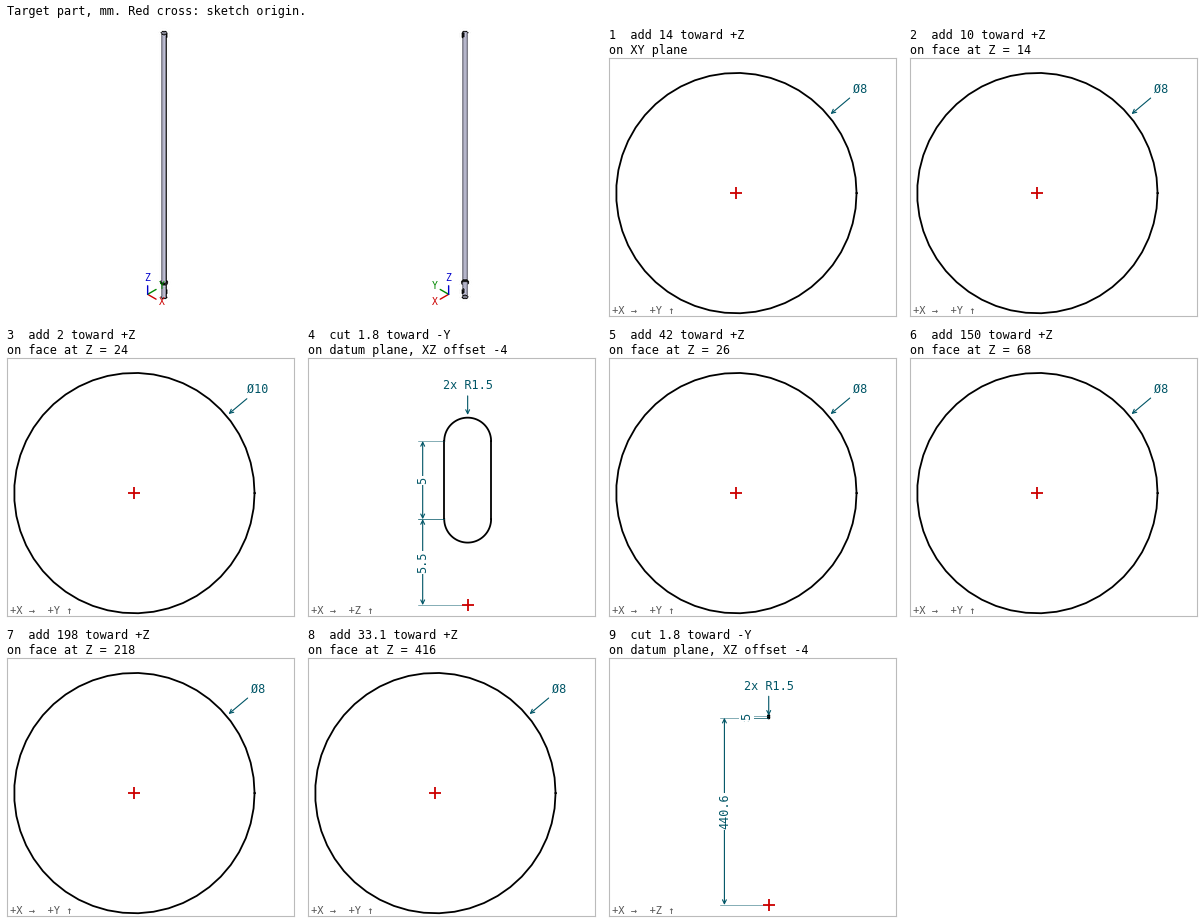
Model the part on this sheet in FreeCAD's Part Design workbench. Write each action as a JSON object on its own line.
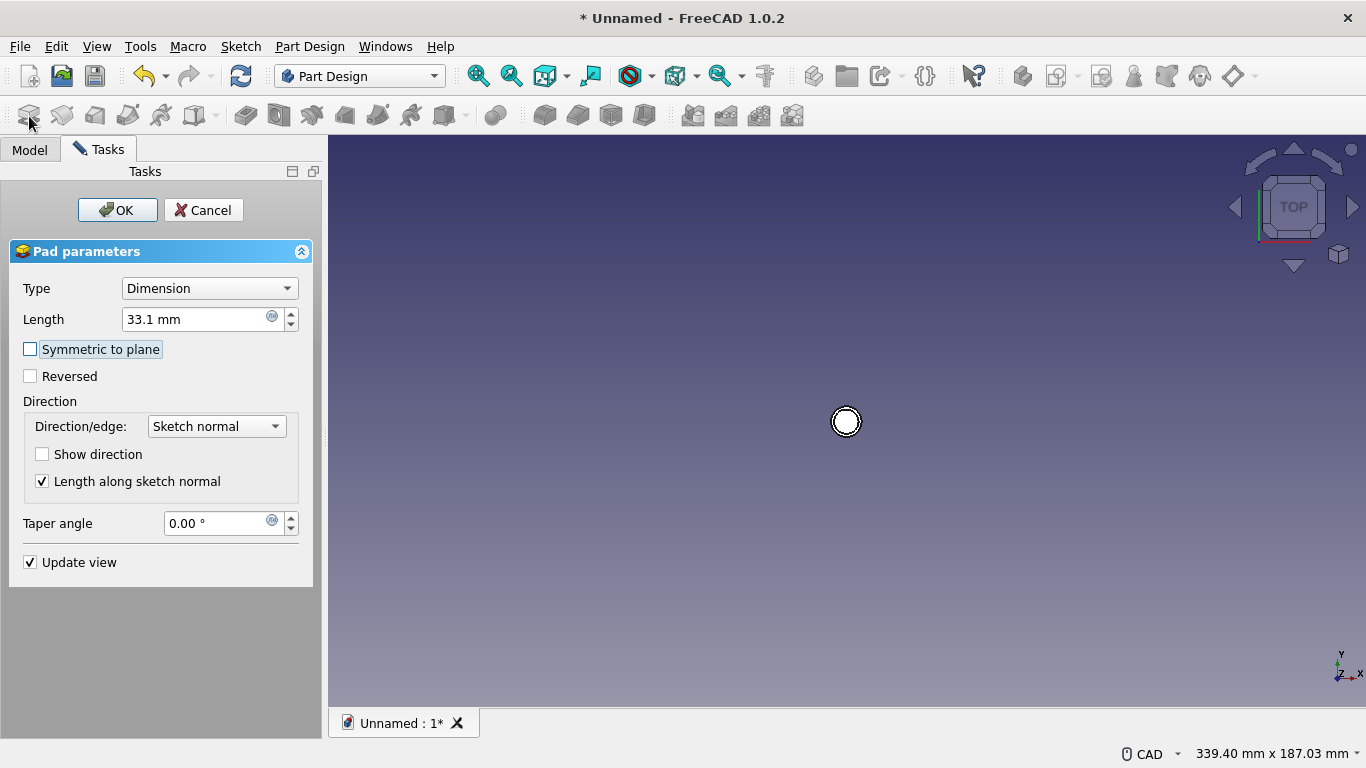
{"action": "left_click", "coordinate": [118, 210]}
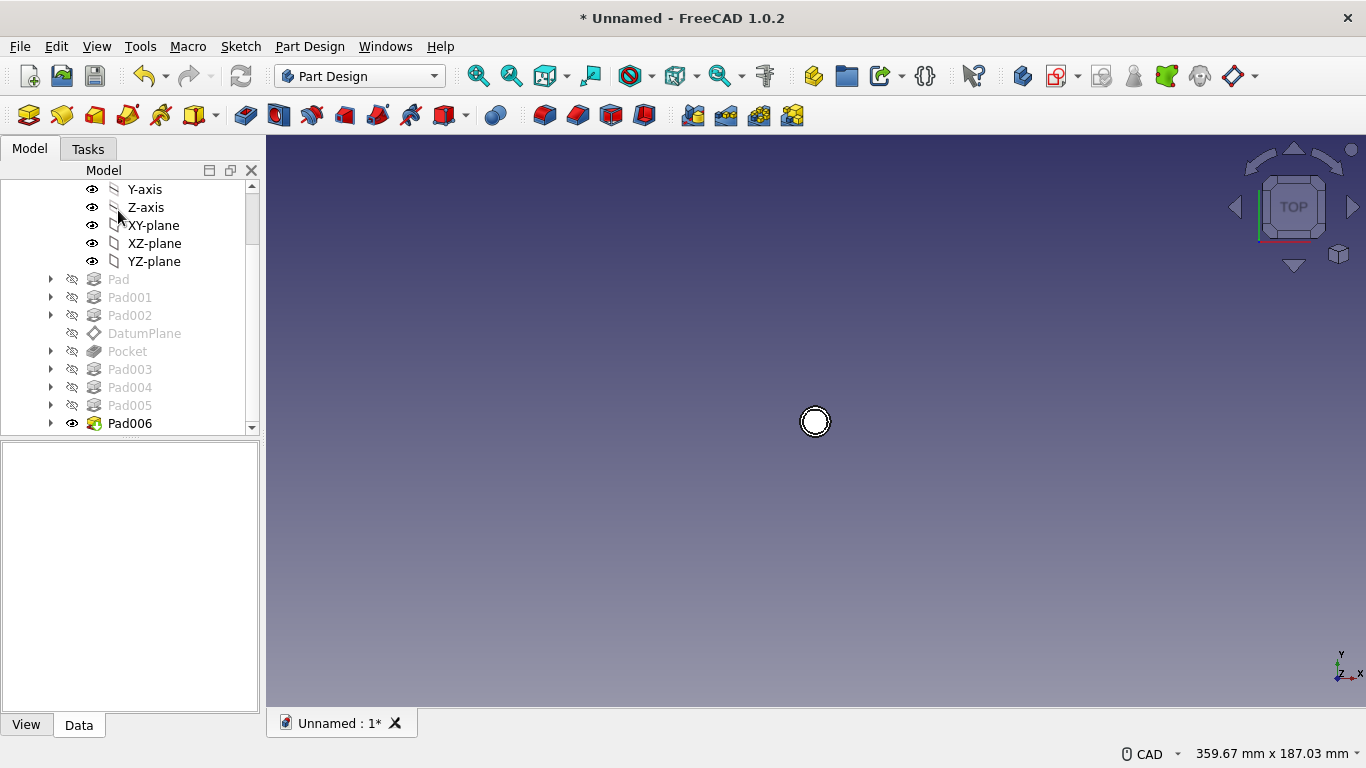
{"action": "left_click", "coordinate": [479, 76]}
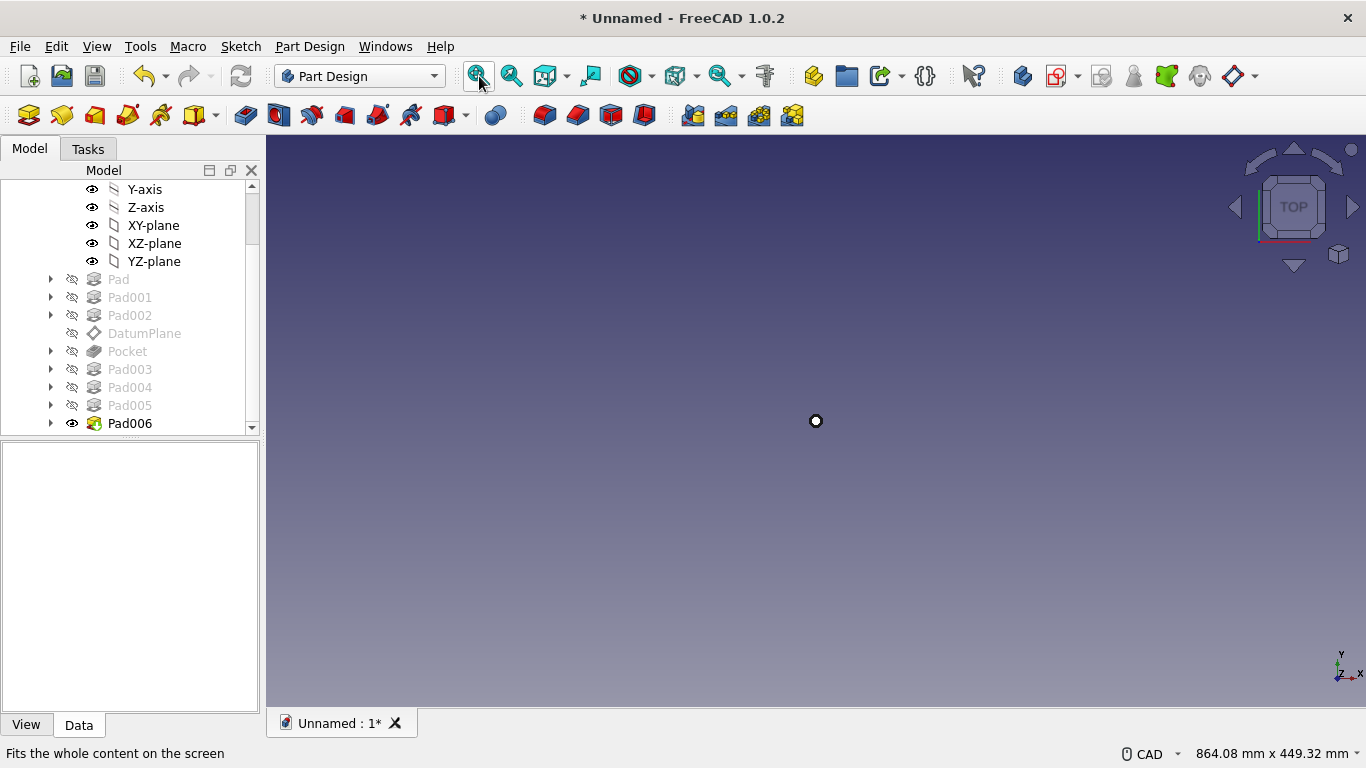
{"action": "scroll", "coordinate": [161, 311], "scroll_direction": "down", "scroll_amount": 3}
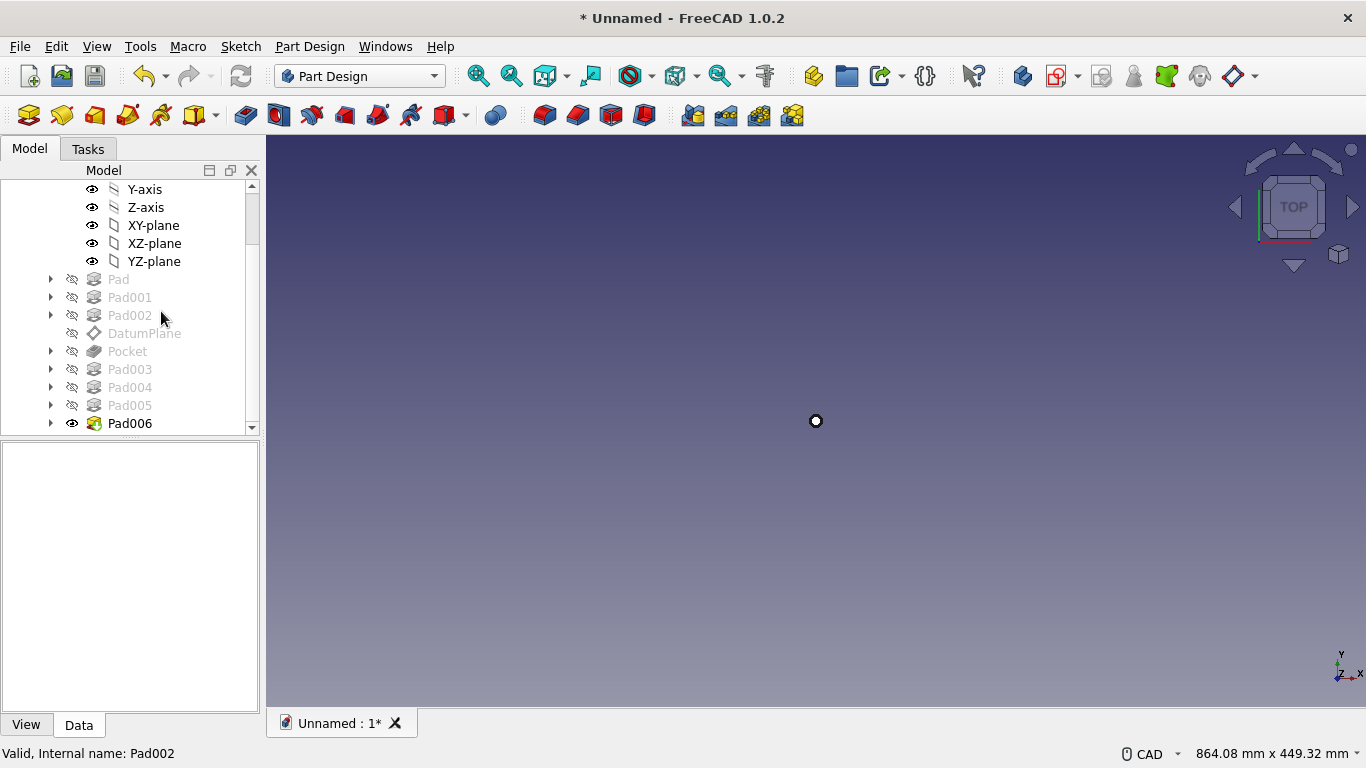
{"action": "scroll", "coordinate": [161, 311], "scroll_direction": "up", "scroll_amount": 15}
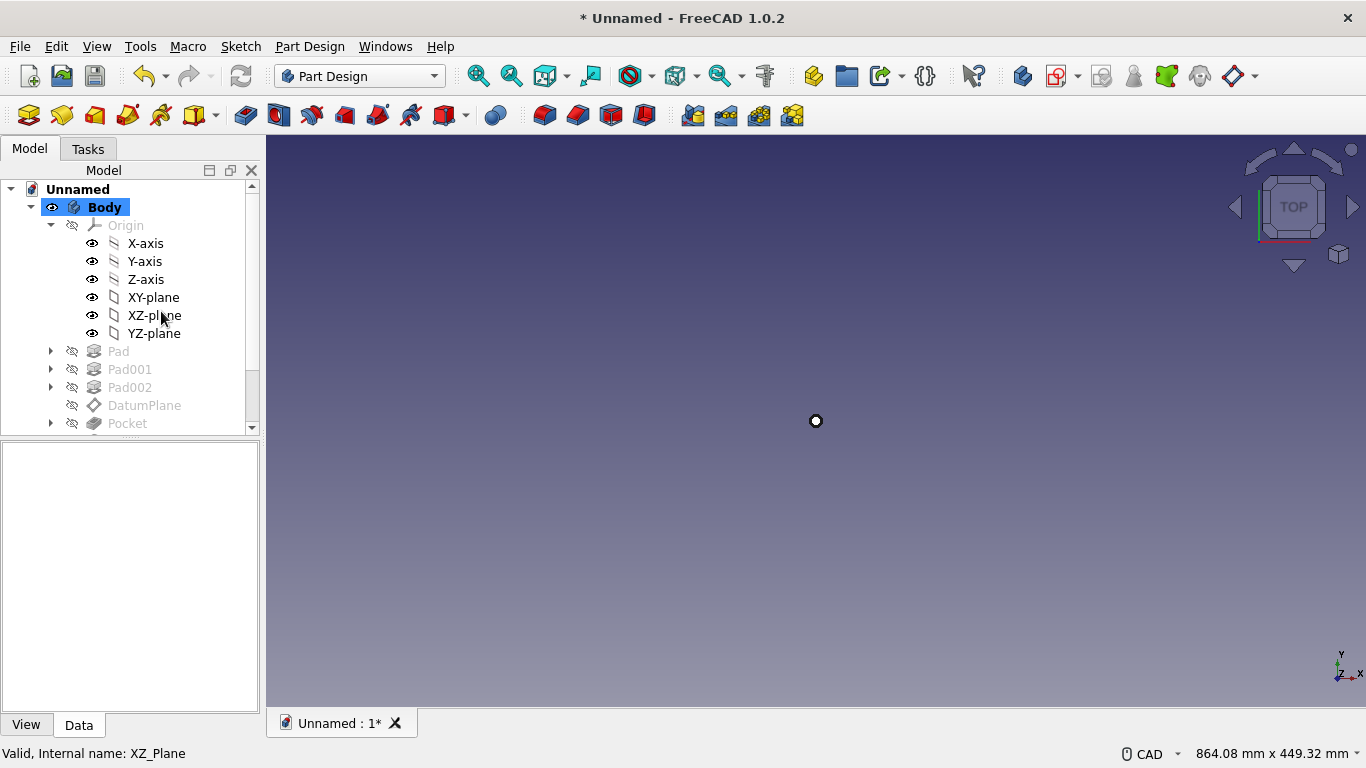
{"action": "left_click", "coordinate": [137, 315]}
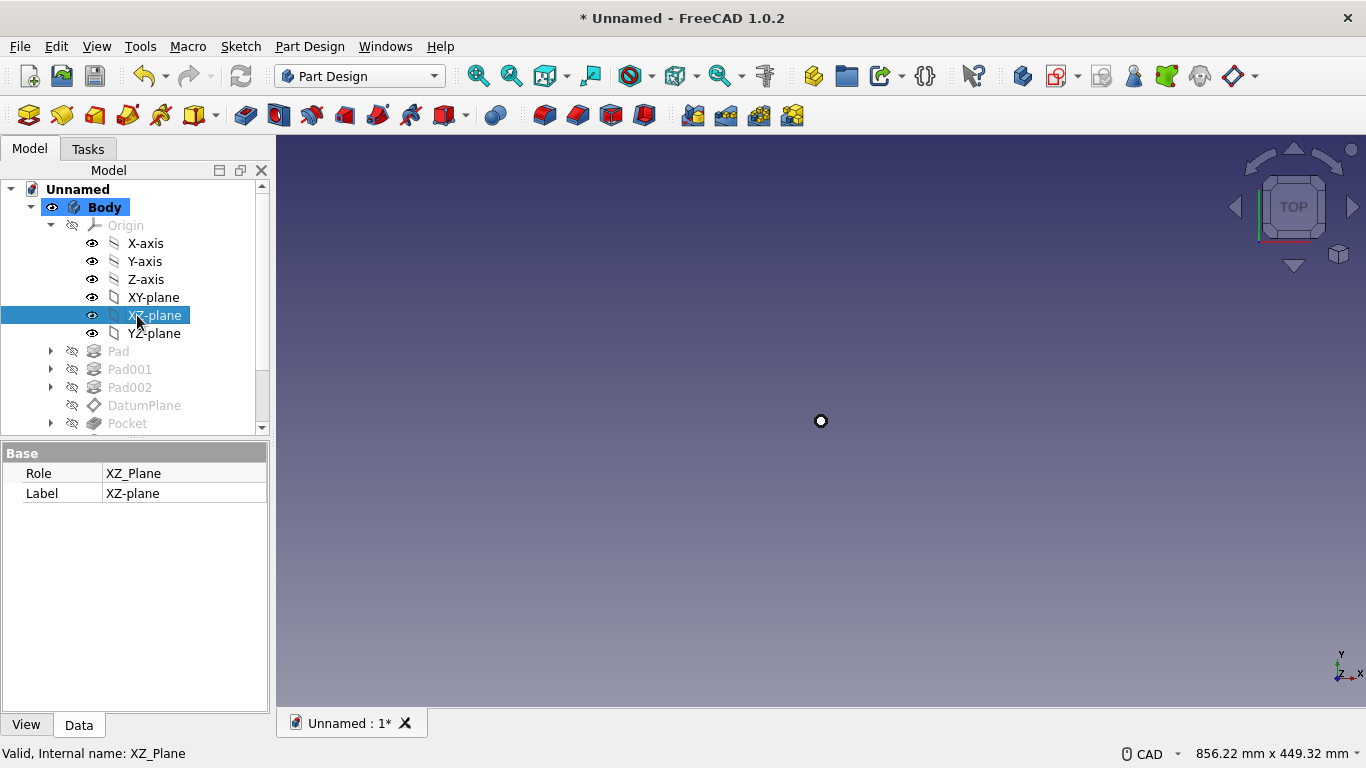
{"action": "left_click", "coordinate": [1232, 76]}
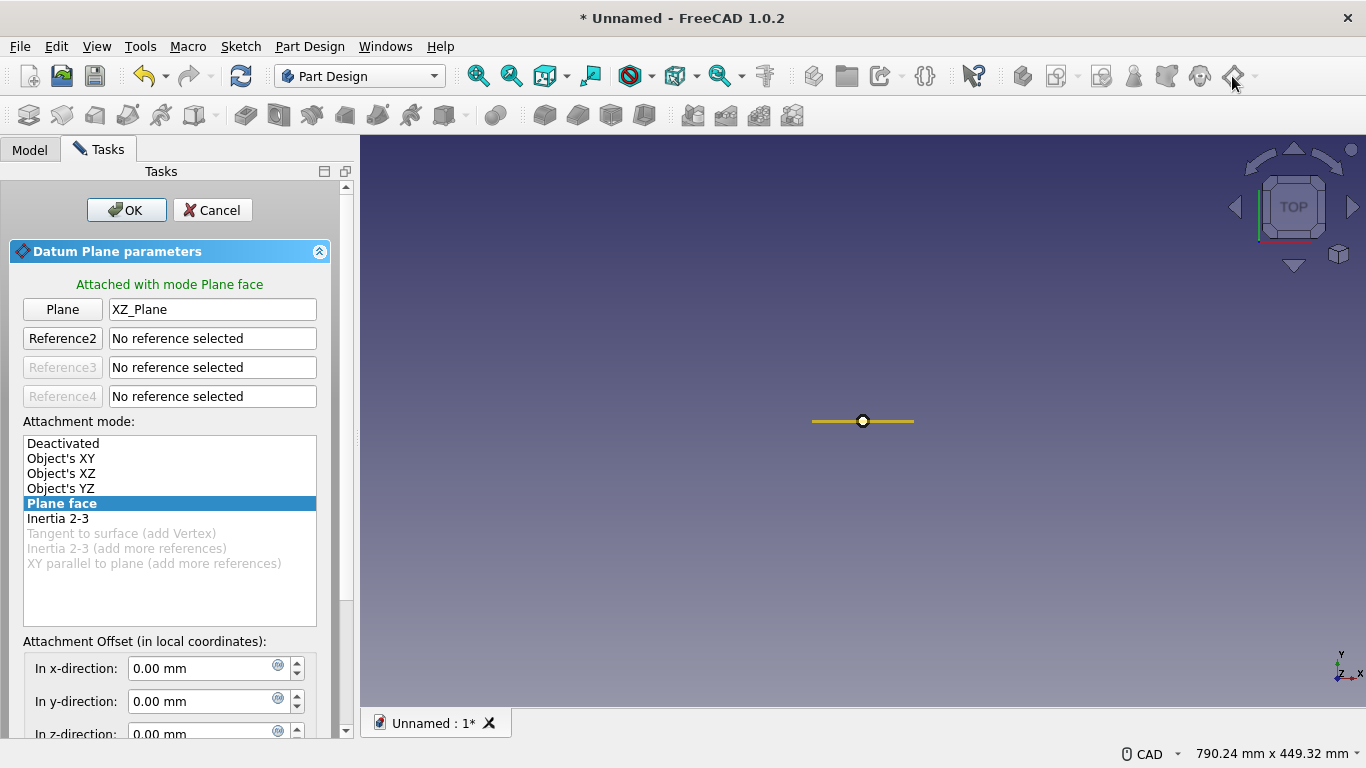
{"action": "scroll", "coordinate": [346, 460], "scroll_direction": "down", "scroll_amount": 2}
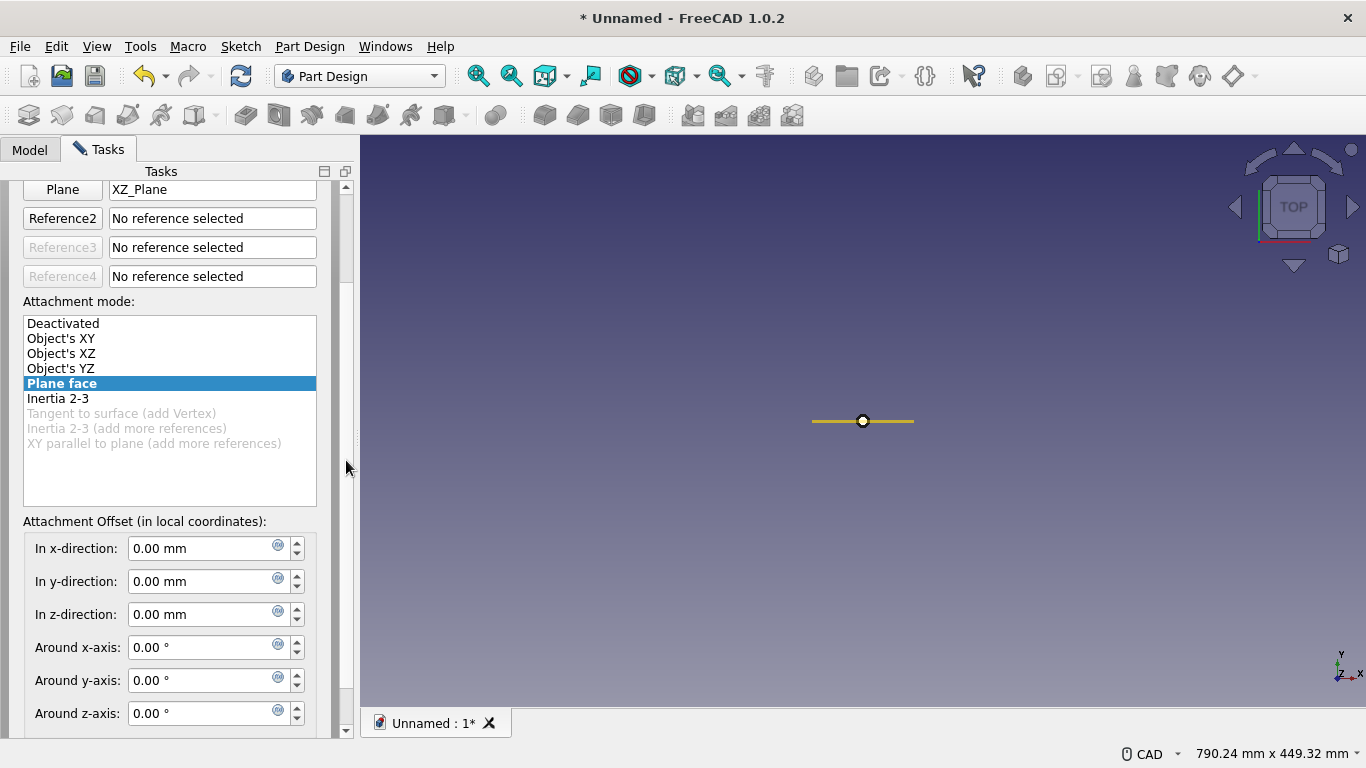
{"action": "triple_click", "coordinate": [210, 614]}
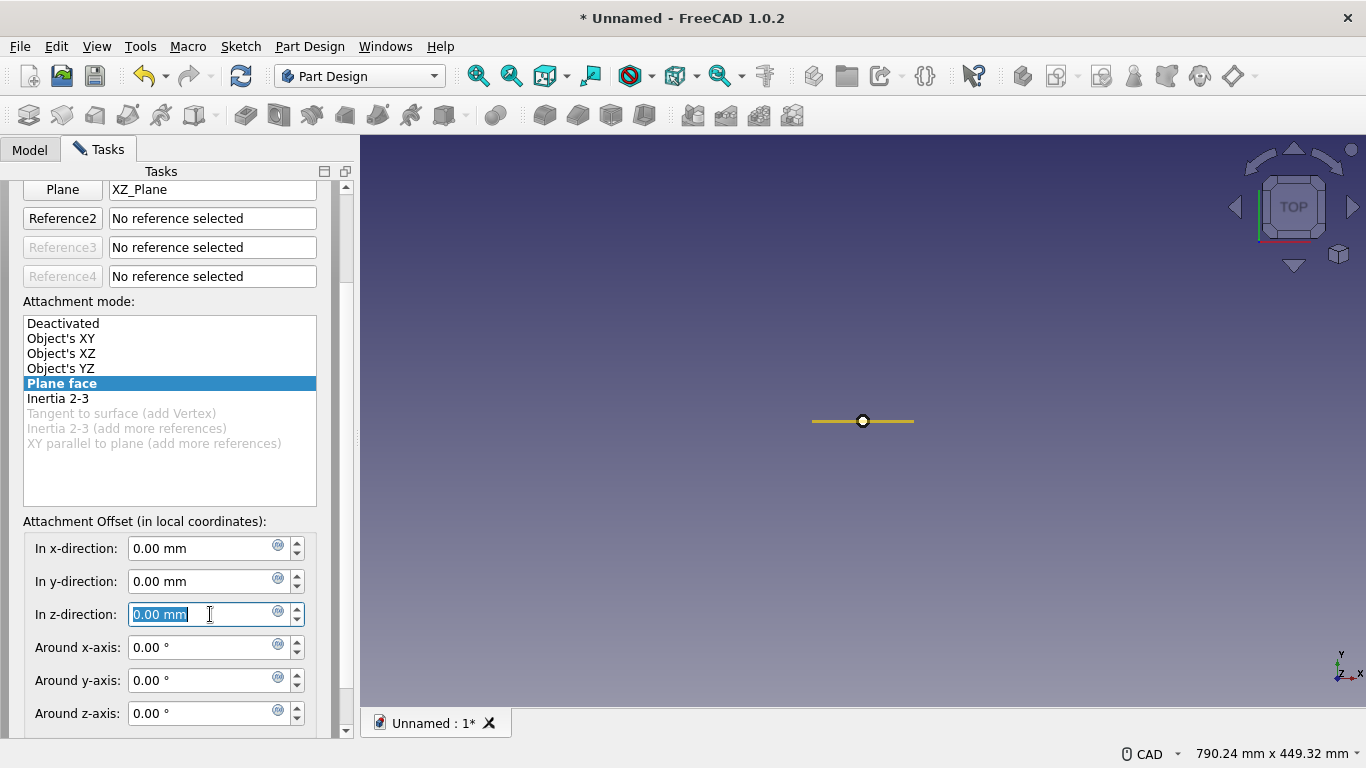
{"action": "type", "text": "-4"}
{"action": "key", "text": "Tab"}